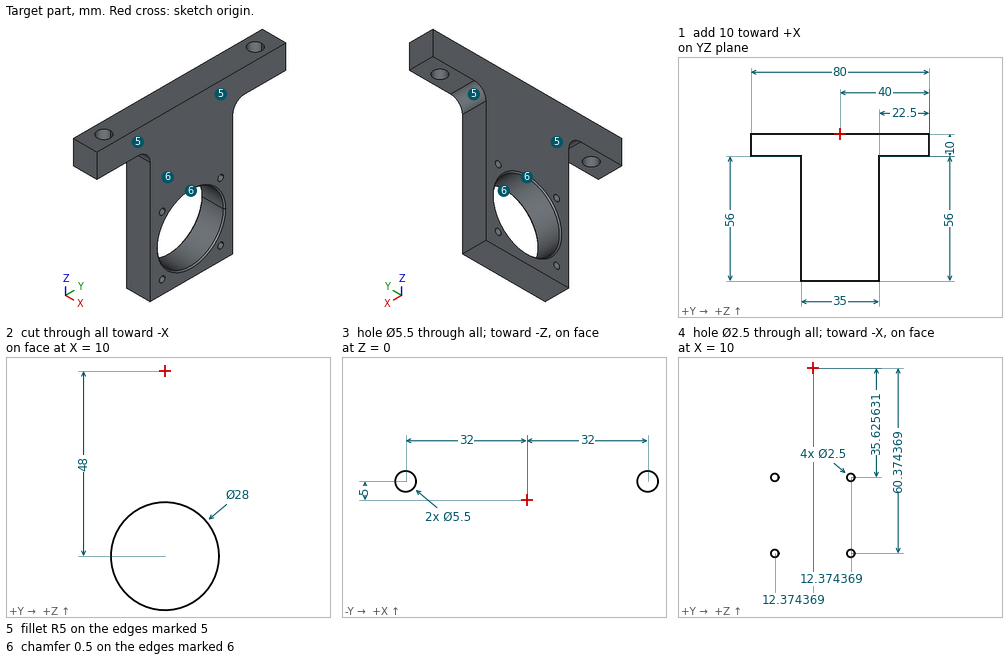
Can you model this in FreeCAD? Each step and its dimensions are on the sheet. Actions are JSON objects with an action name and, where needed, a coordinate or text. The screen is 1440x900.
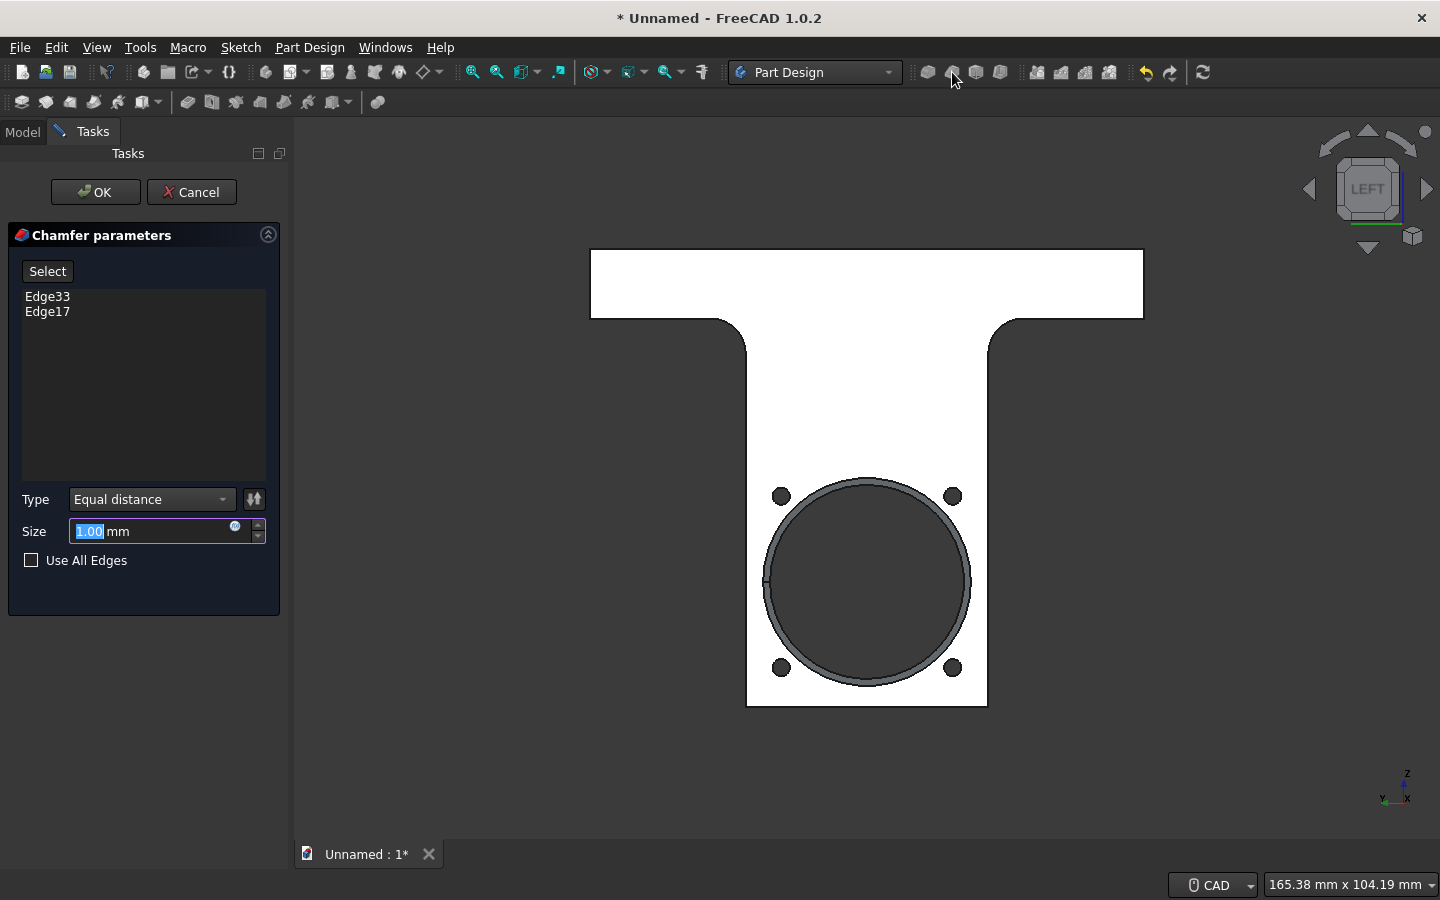
{"action": "type", "text": "0.5"}
{"action": "key", "text": "Tab"}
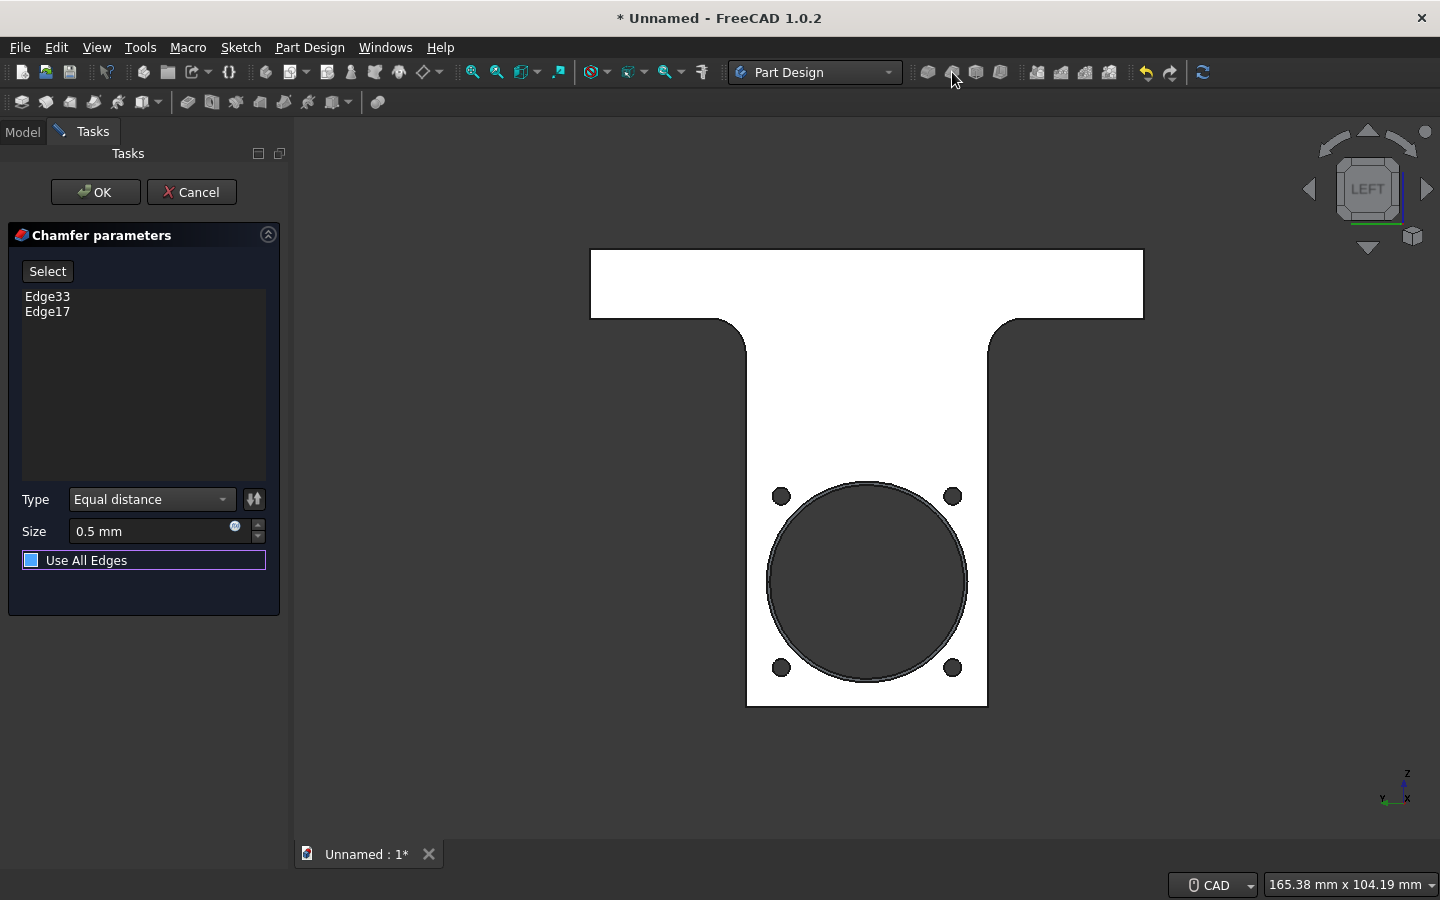
{"action": "left_click", "coordinate": [96, 192]}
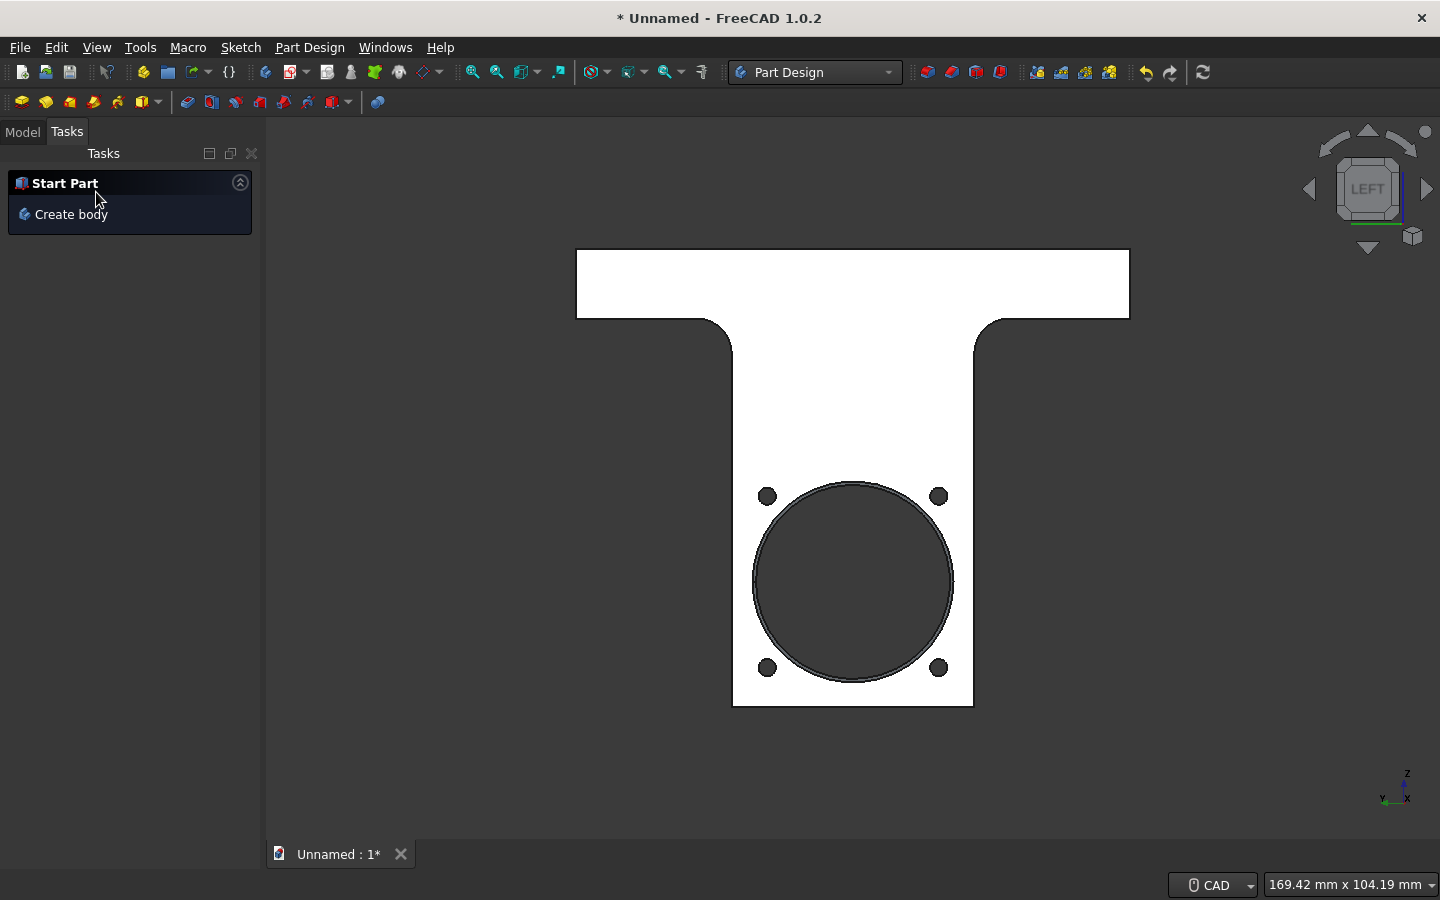
{"action": "key", "text": "0"}